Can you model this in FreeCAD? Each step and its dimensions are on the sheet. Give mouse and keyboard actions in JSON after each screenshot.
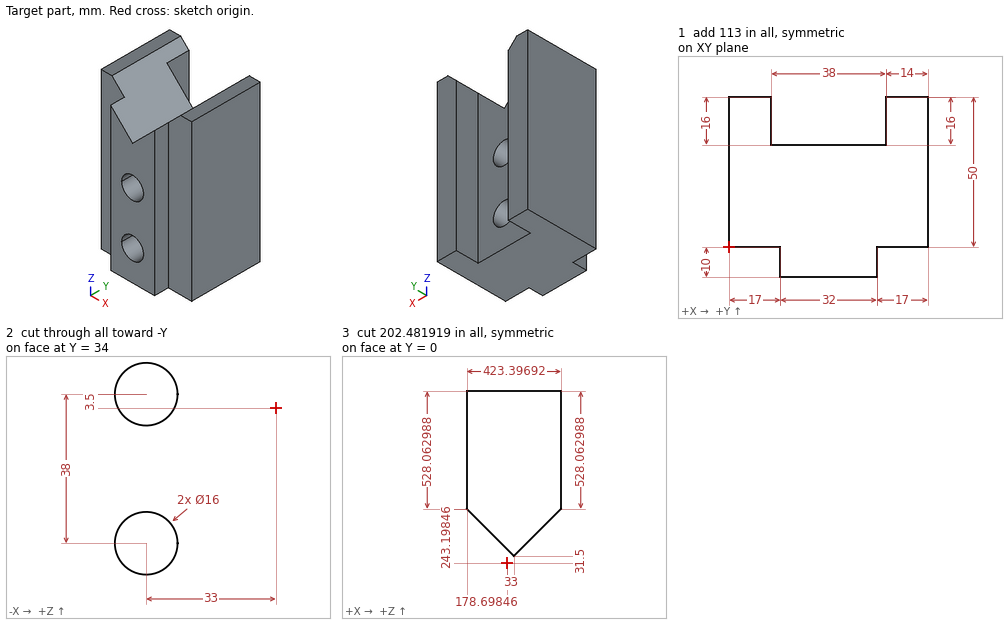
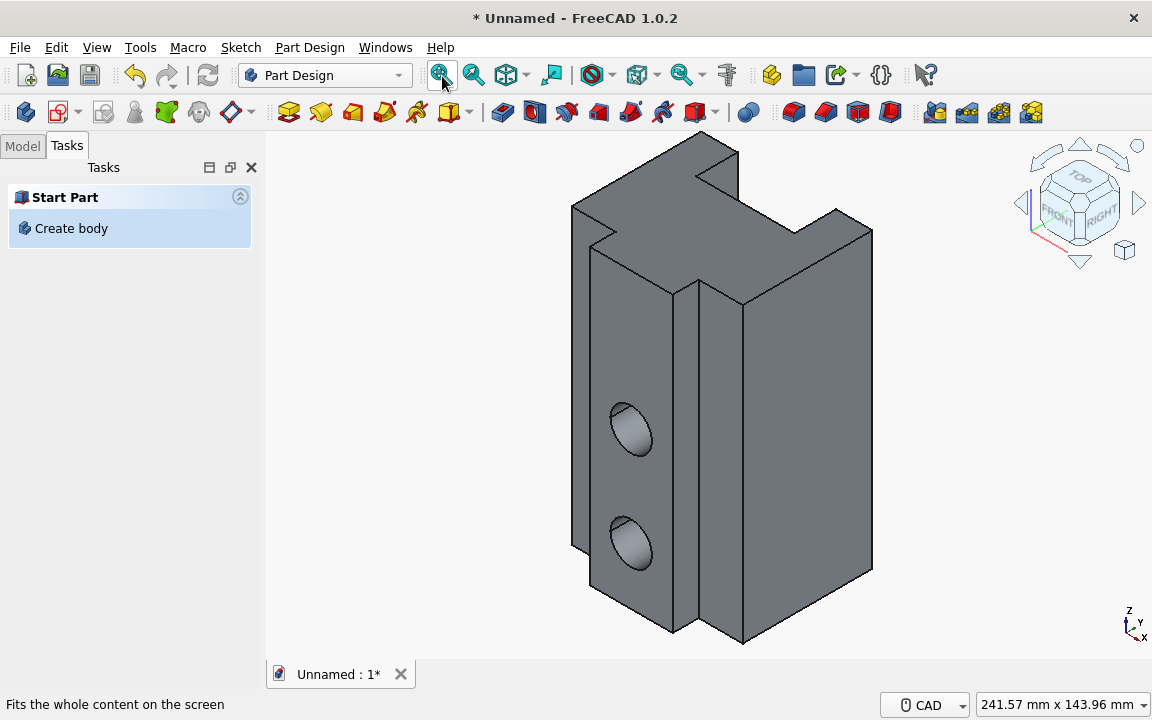
{"action": "left_click", "coordinate": [721, 364]}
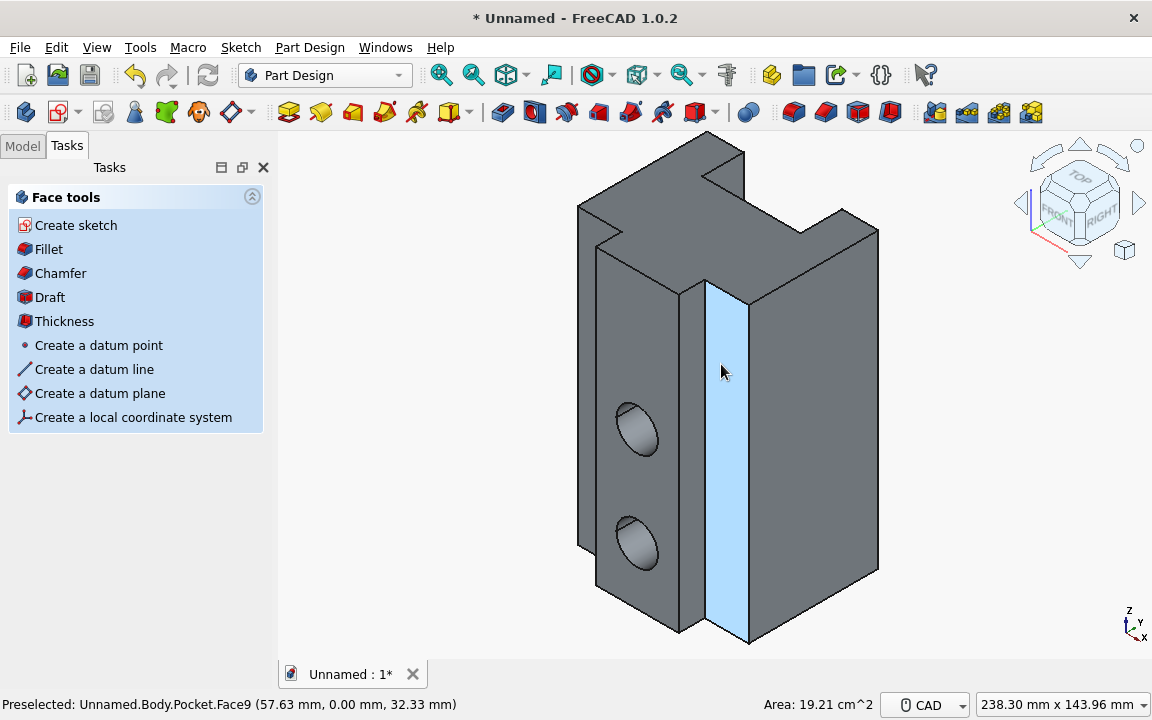
{"action": "left_click", "coordinate": [58, 112]}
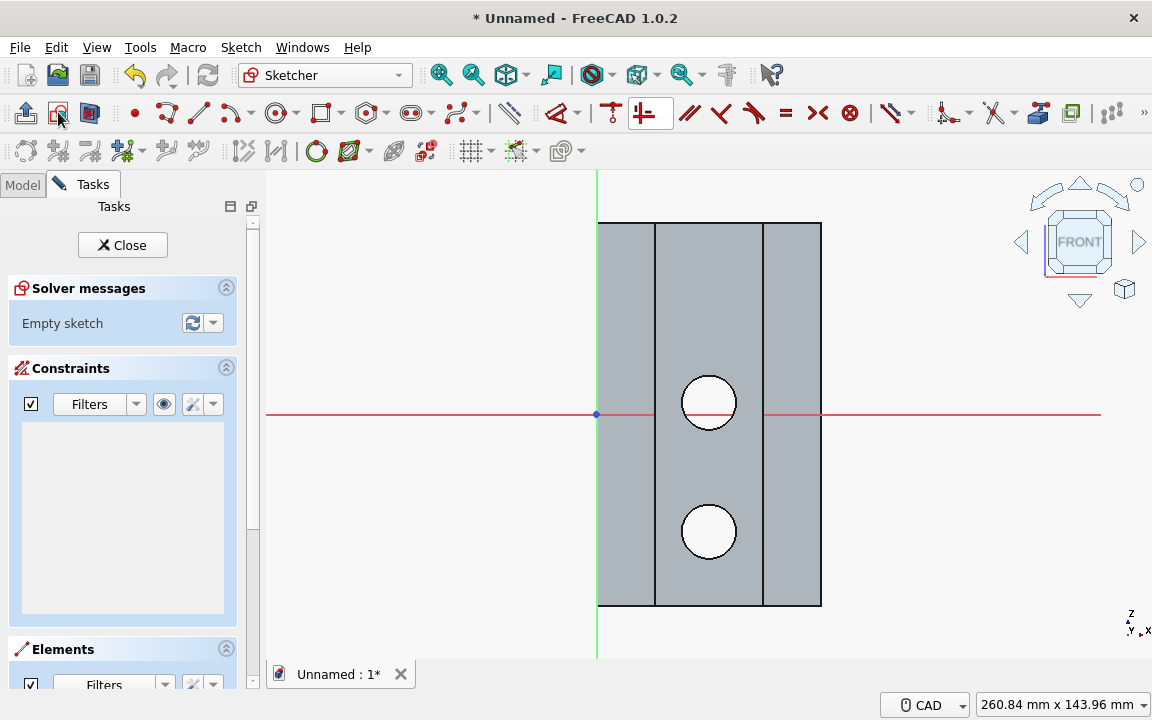
{"action": "left_click", "coordinate": [90, 114]}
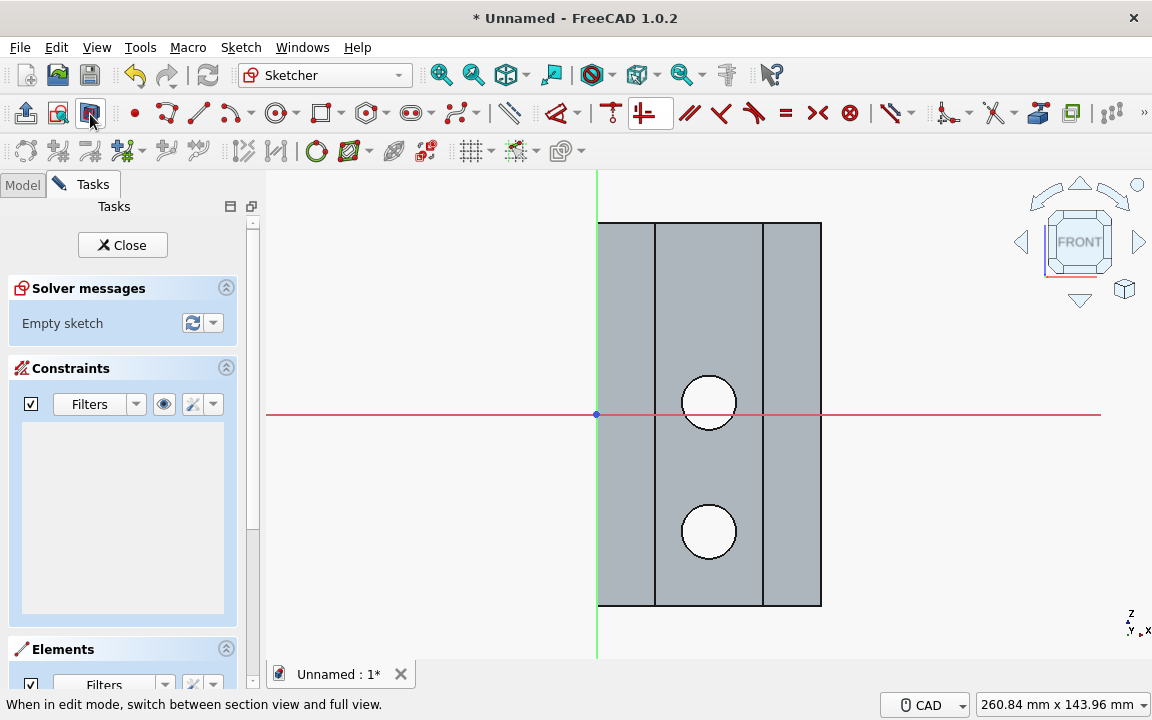
{"action": "scroll", "coordinate": [632, 578], "scroll_direction": "down", "scroll_amount": 11}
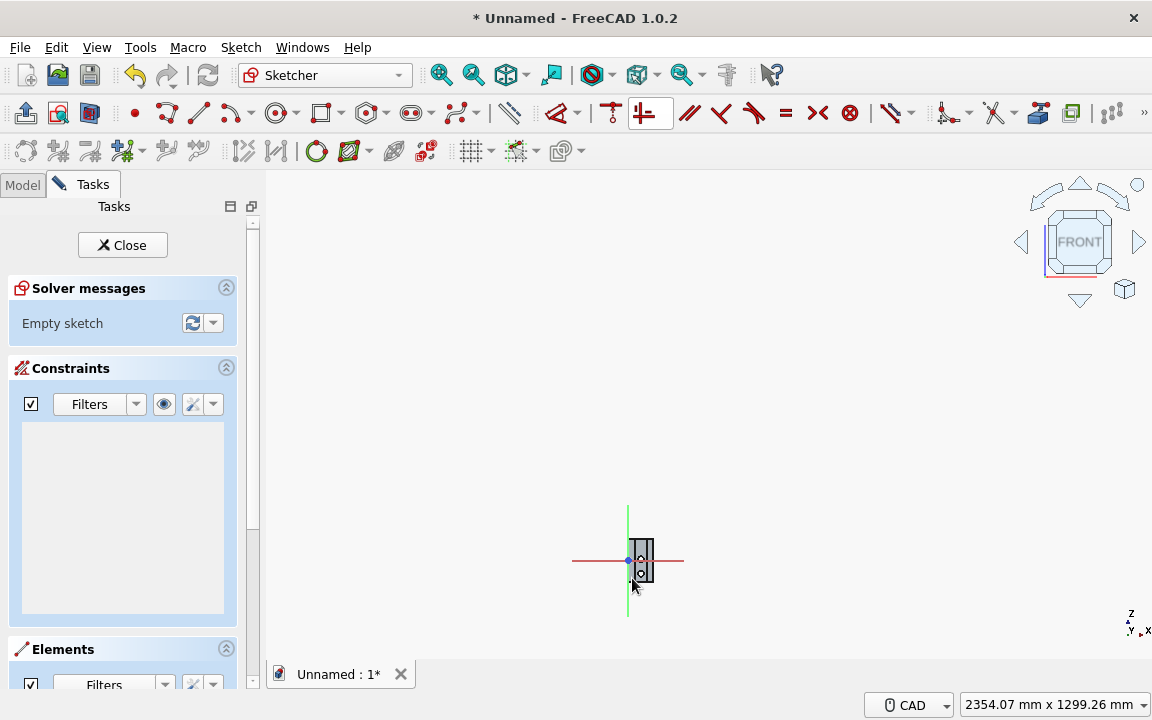
{"action": "left_click", "coordinate": [168, 114]}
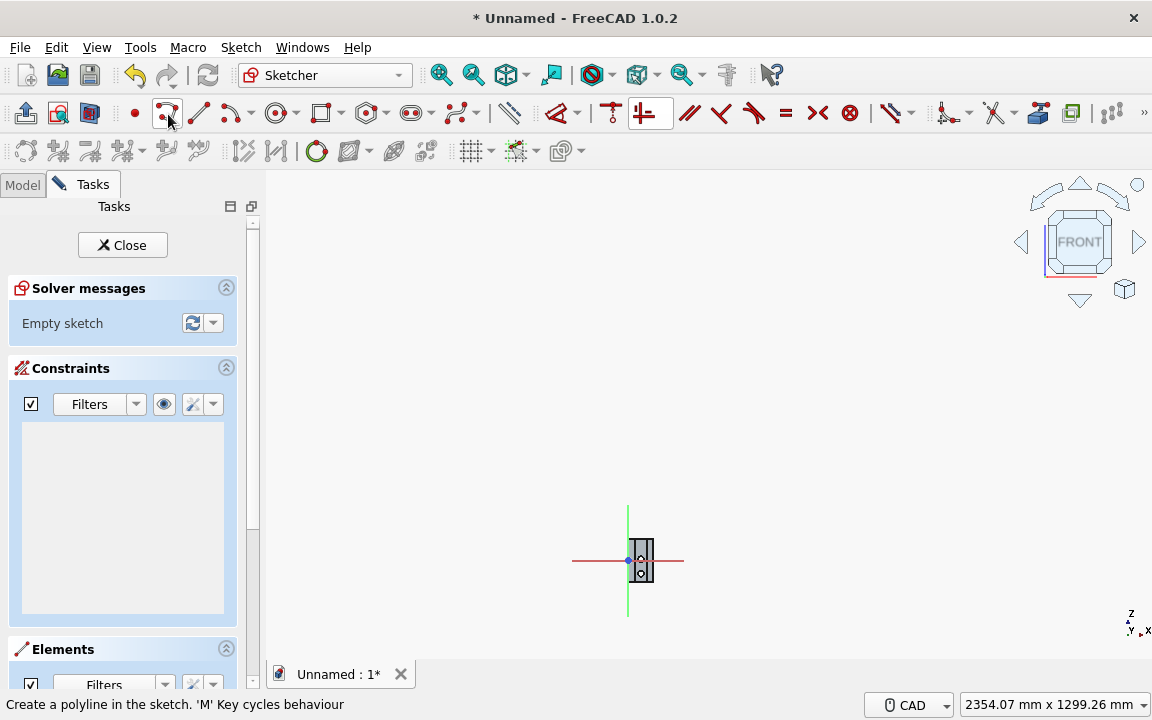
{"action": "scroll", "coordinate": [641, 549], "scroll_direction": "up", "scroll_amount": 2}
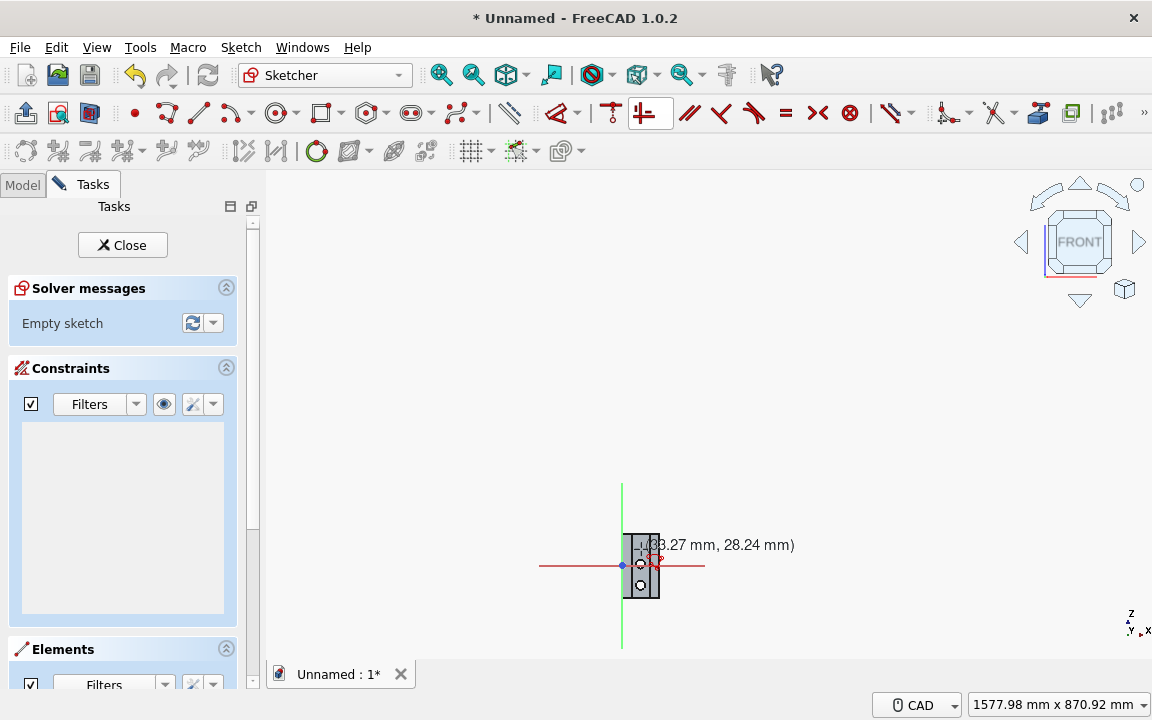
{"action": "left_click", "coordinate": [641, 548]}
{"action": "left_click", "coordinate": [522, 429]}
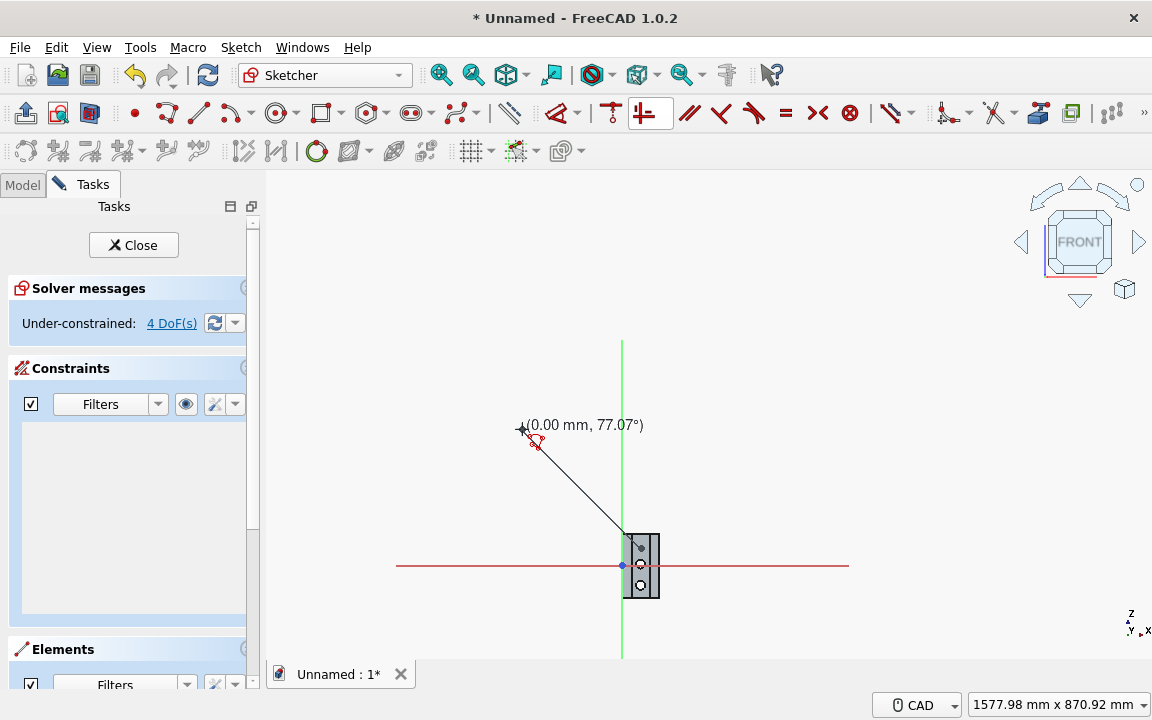
{"action": "scroll", "coordinate": [640, 547], "scroll_direction": "down", "scroll_amount": 2}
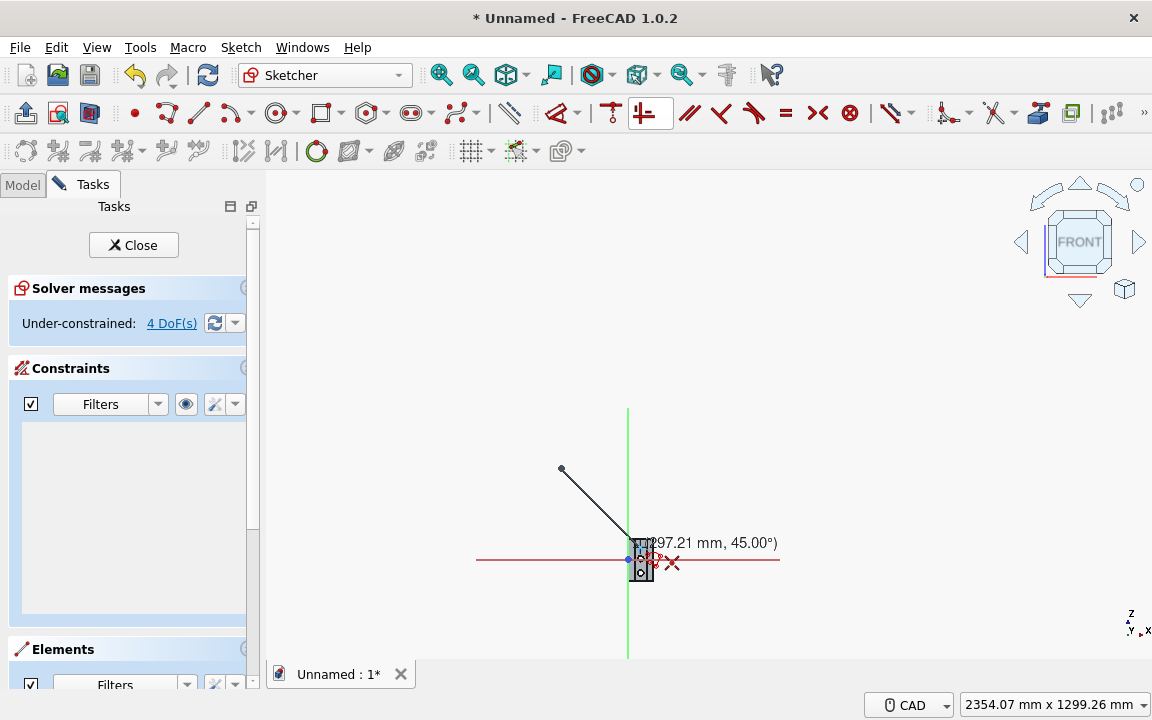
{"action": "left_click", "coordinate": [561, 270]}
{"action": "left_click", "coordinate": [720, 270]}
{"action": "left_click", "coordinate": [720, 468]}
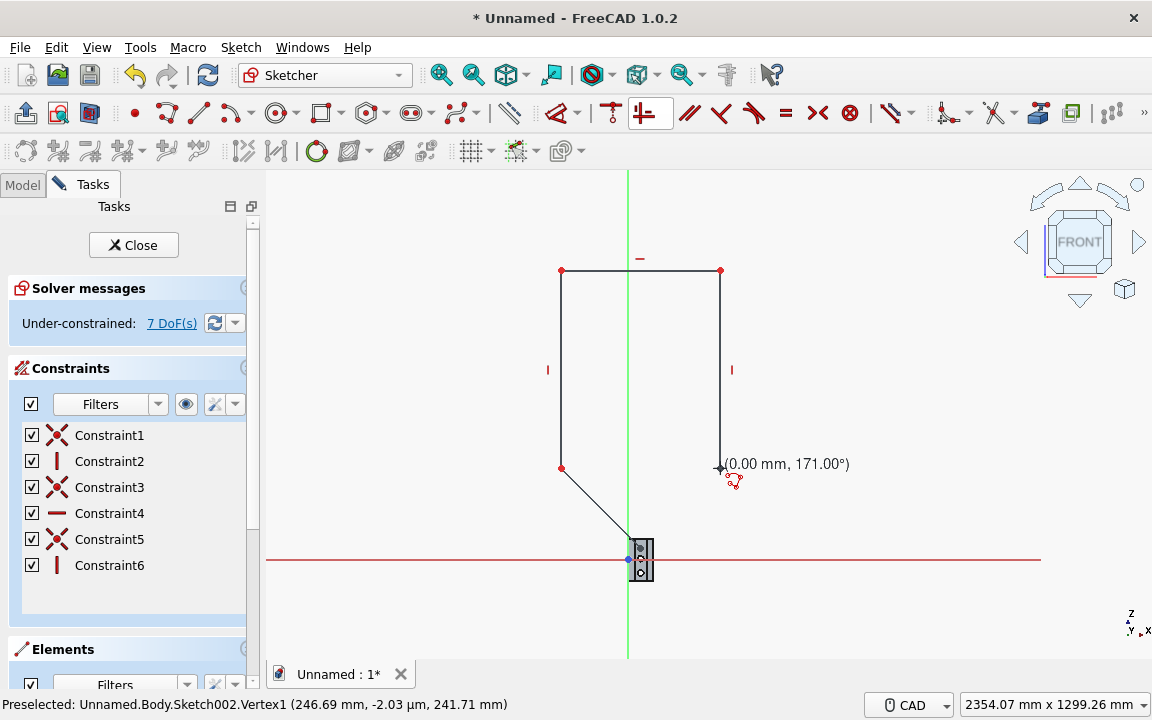
{"action": "scroll", "coordinate": [641, 548], "scroll_direction": "up", "scroll_amount": 2}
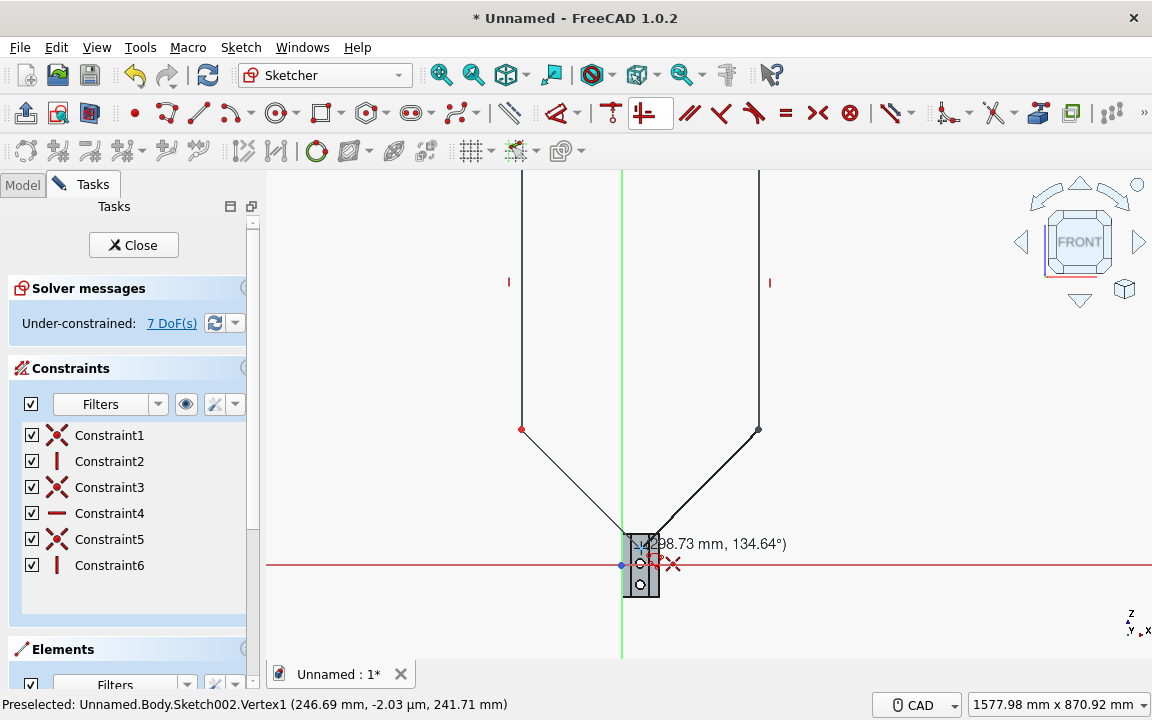
{"action": "left_click", "coordinate": [641, 549]}
{"action": "key", "text": "Escape"}
{"action": "key", "text": "Escape"}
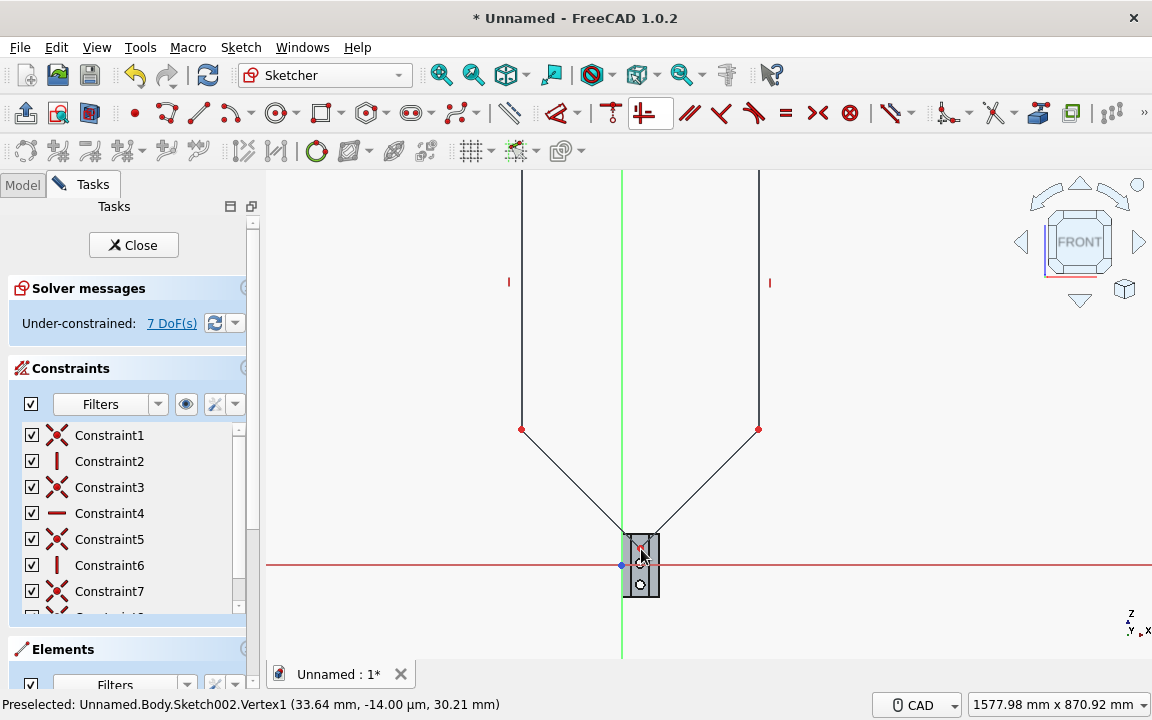
{"action": "left_click", "coordinate": [556, 114]}